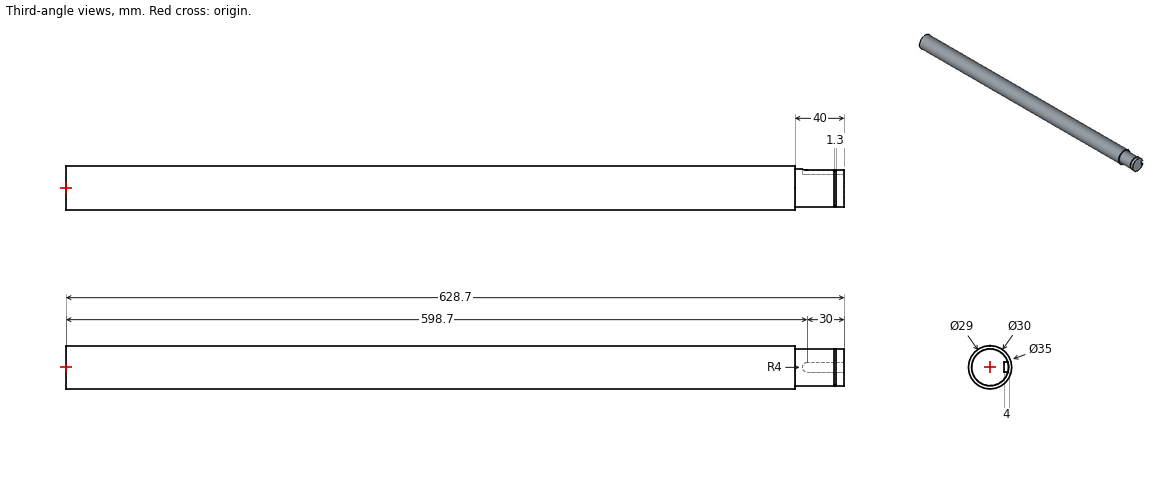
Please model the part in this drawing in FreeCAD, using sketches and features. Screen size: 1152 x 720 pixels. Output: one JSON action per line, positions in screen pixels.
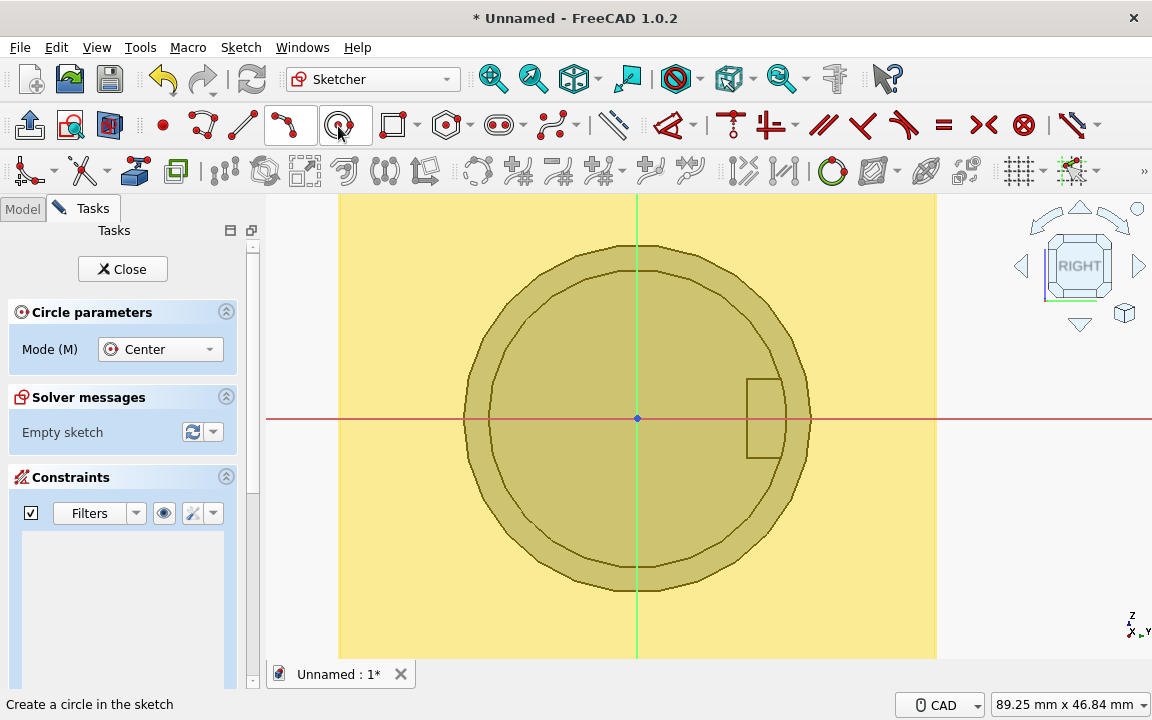
{"action": "left_click", "coordinate": [637, 419]}
{"action": "left_click", "coordinate": [743, 313]}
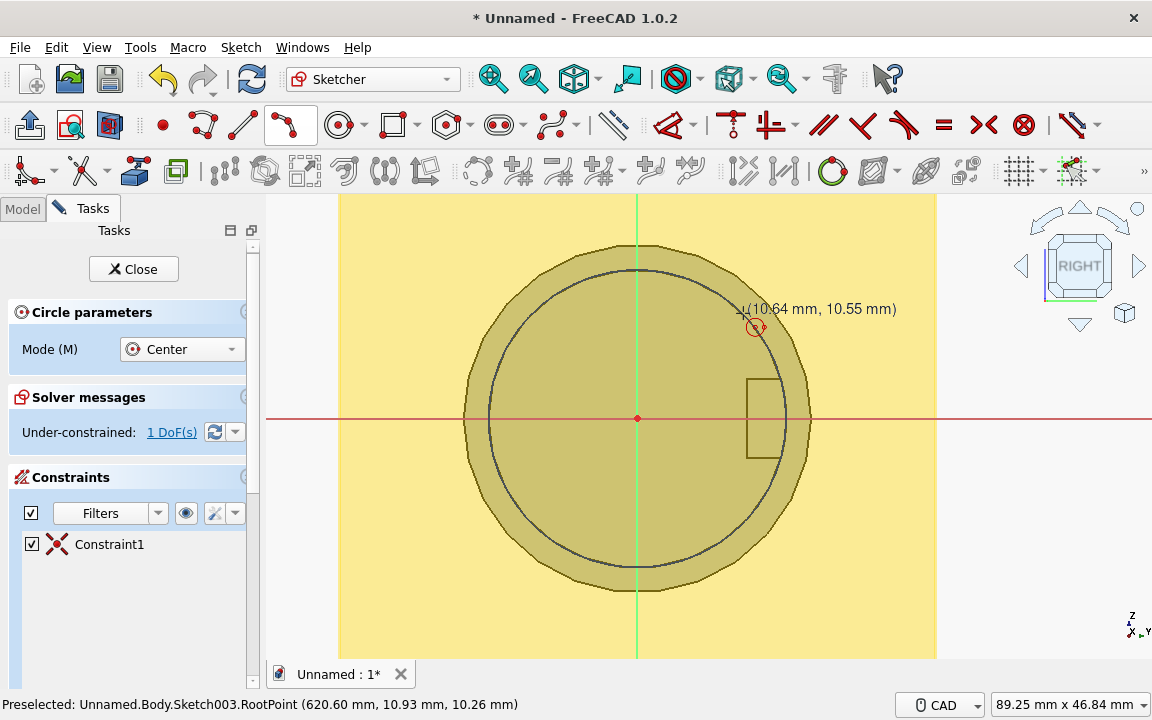
{"action": "left_click", "coordinate": [637, 419]}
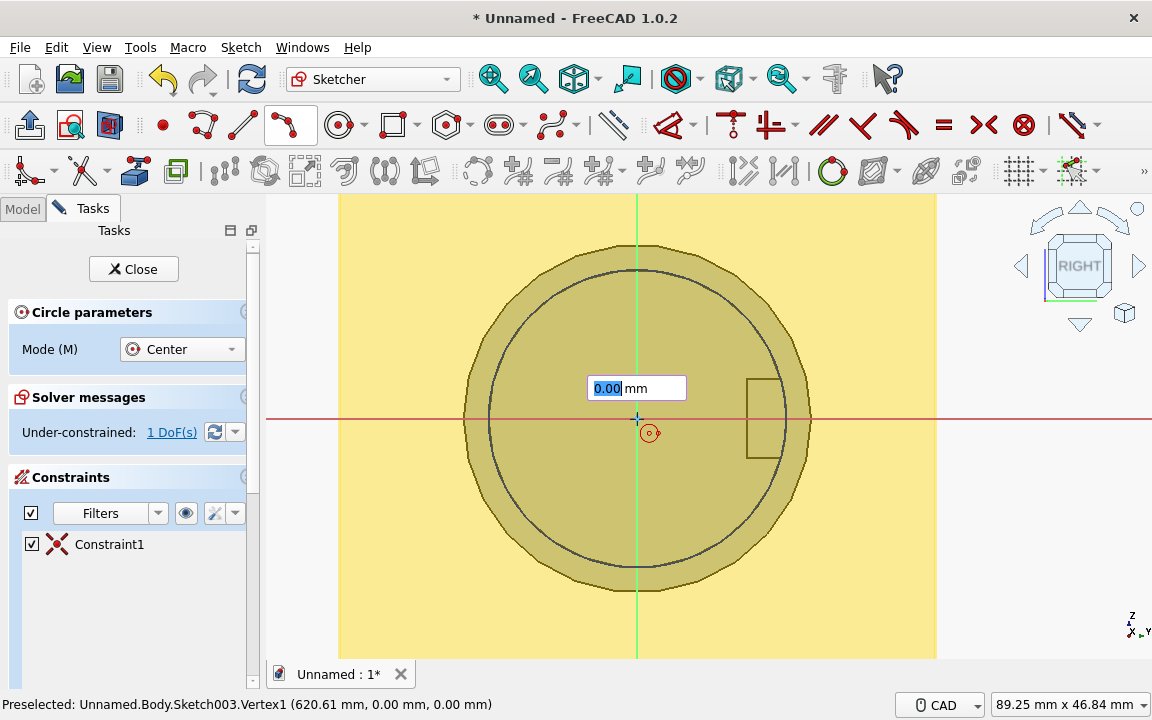
{"action": "scroll", "coordinate": [687, 284], "scroll_direction": "up", "scroll_amount": 6}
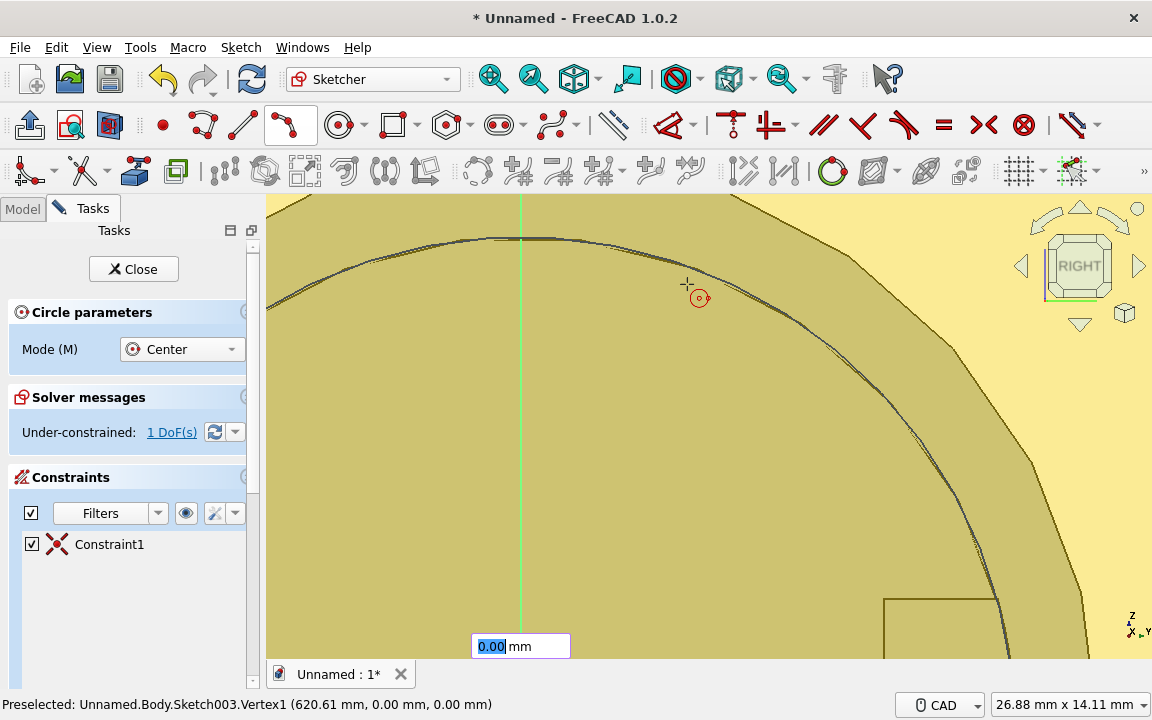
{"action": "left_click", "coordinate": [685, 282]}
{"action": "key", "text": "Escape"}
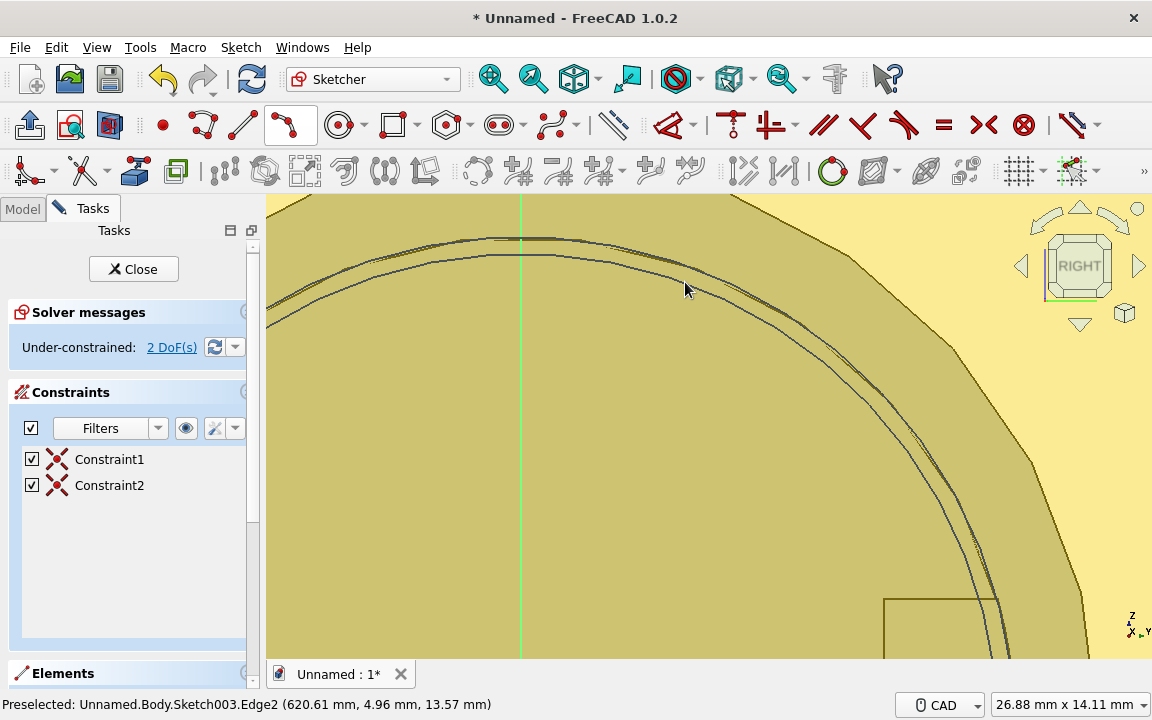
{"action": "left_click", "coordinate": [668, 126]}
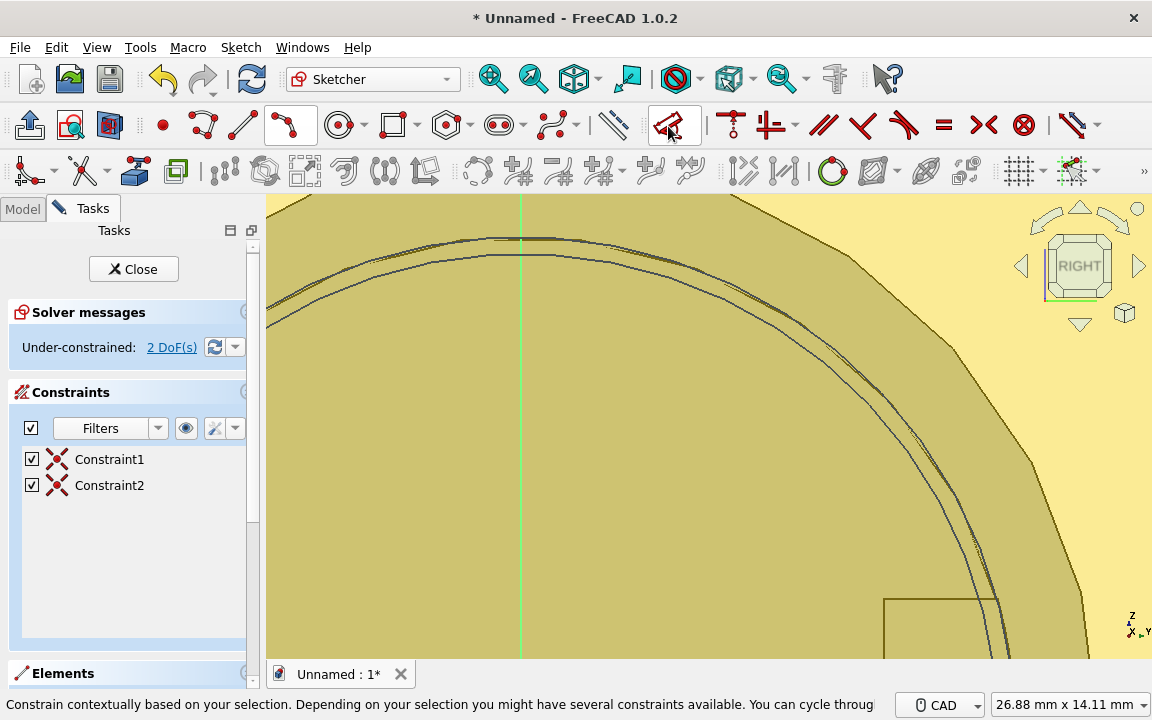
{"action": "left_click", "coordinate": [869, 381]}
{"action": "left_click", "coordinate": [892, 358]}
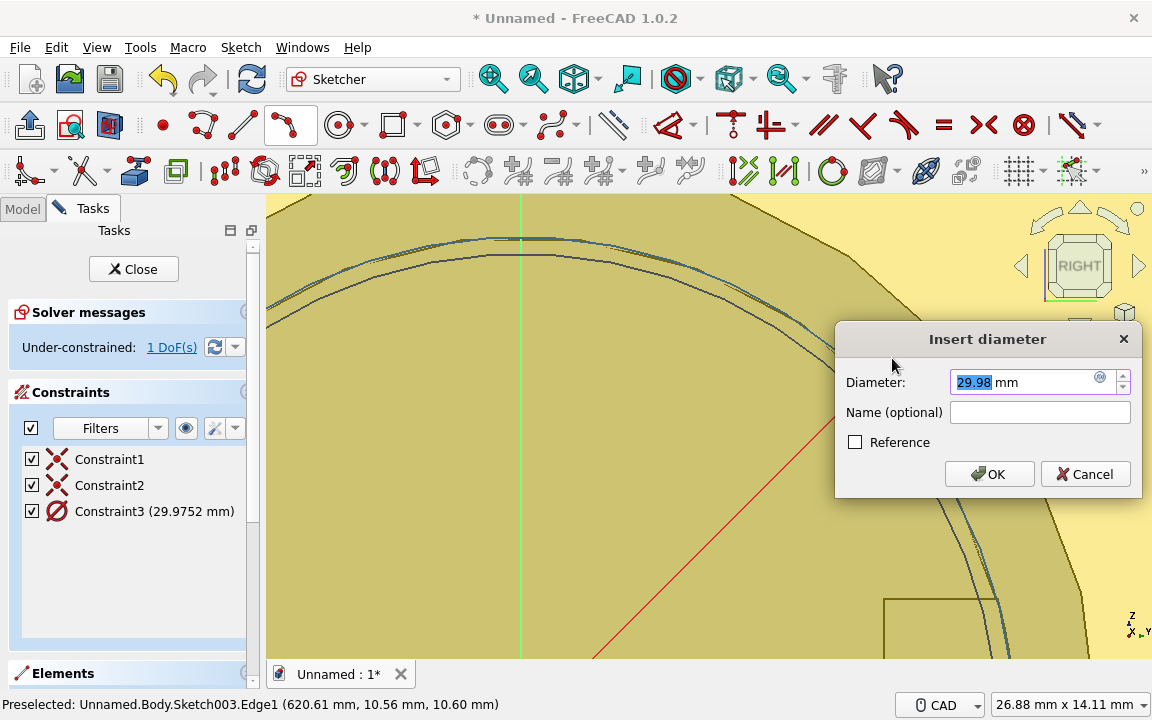
{"action": "type", "text": "30"}
{"action": "key", "text": "Return"}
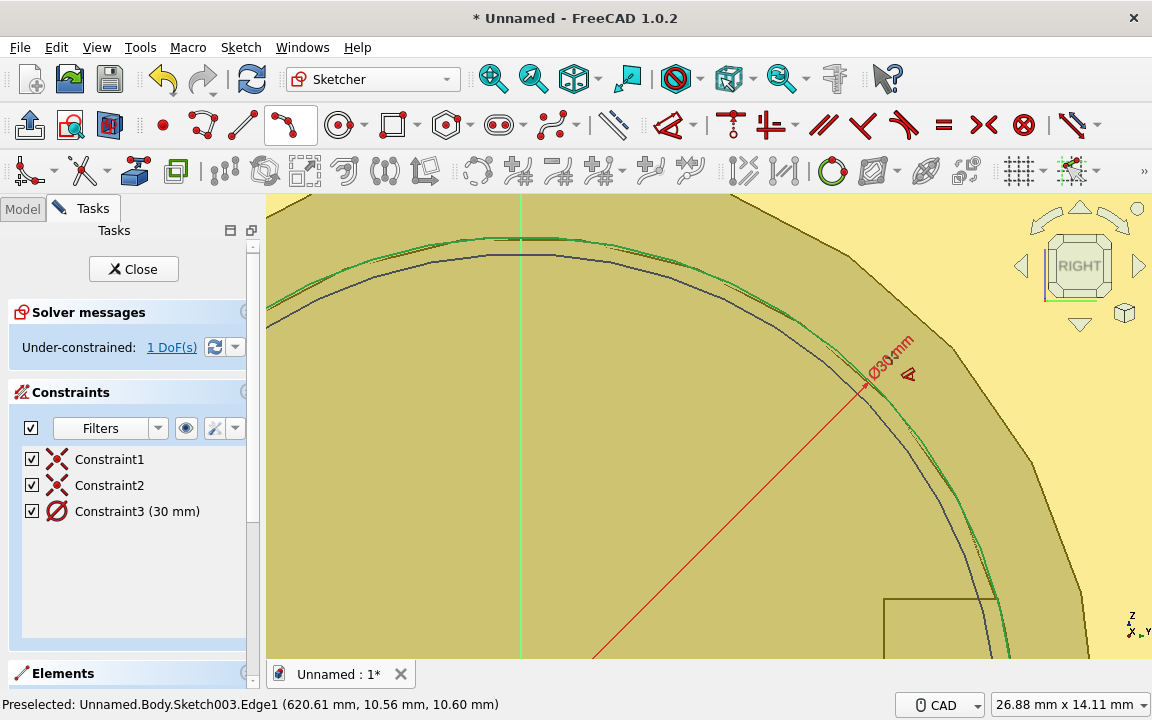
{"action": "left_click", "coordinate": [857, 393]}
{"action": "left_click", "coordinate": [663, 243]}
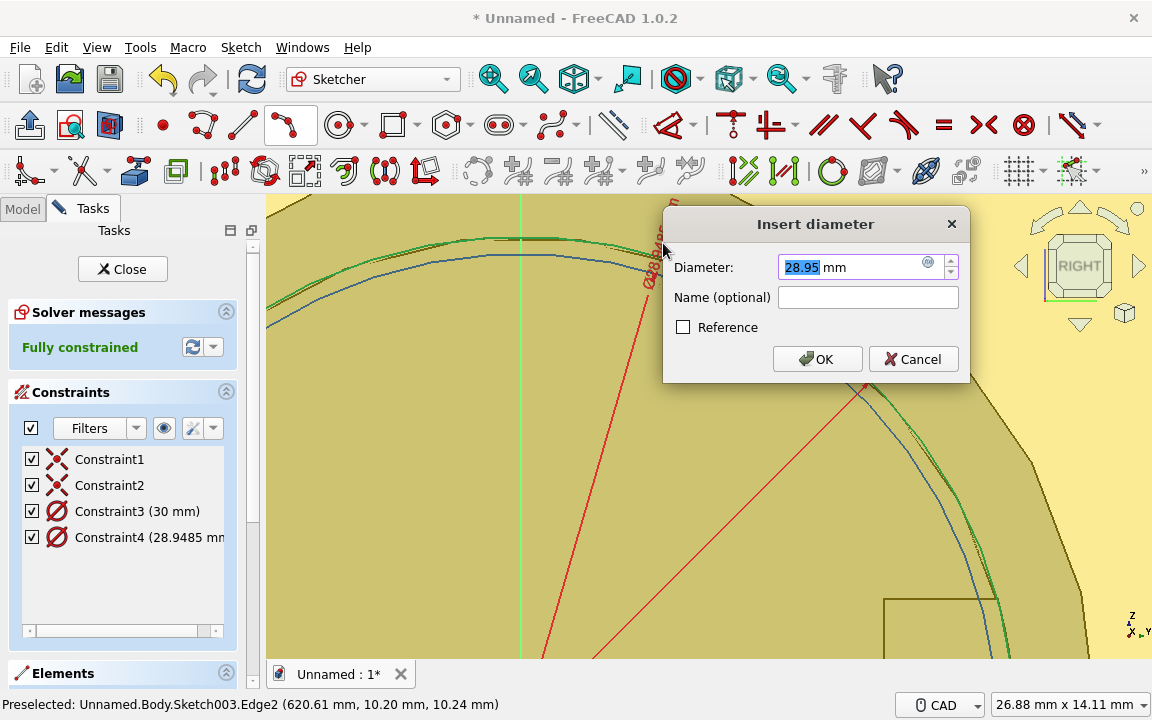
{"action": "type", "text": "29"}
{"action": "key", "text": "Return"}
{"action": "key", "text": "Escape"}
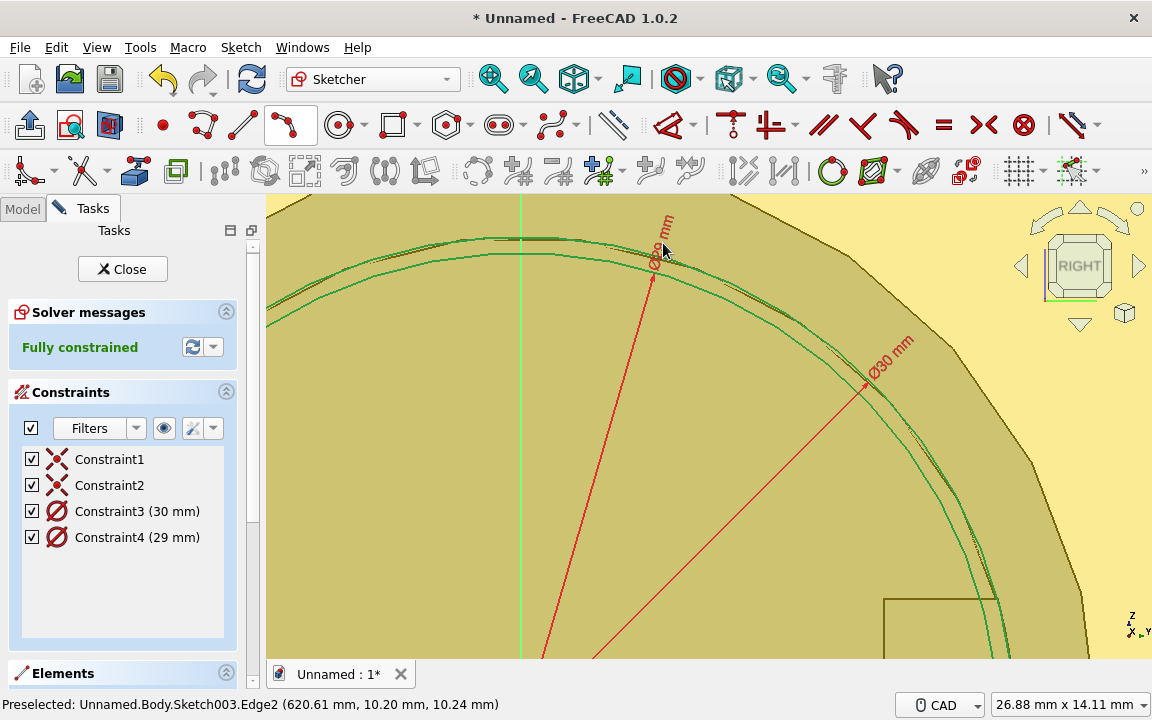
{"action": "left_click", "coordinate": [123, 269]}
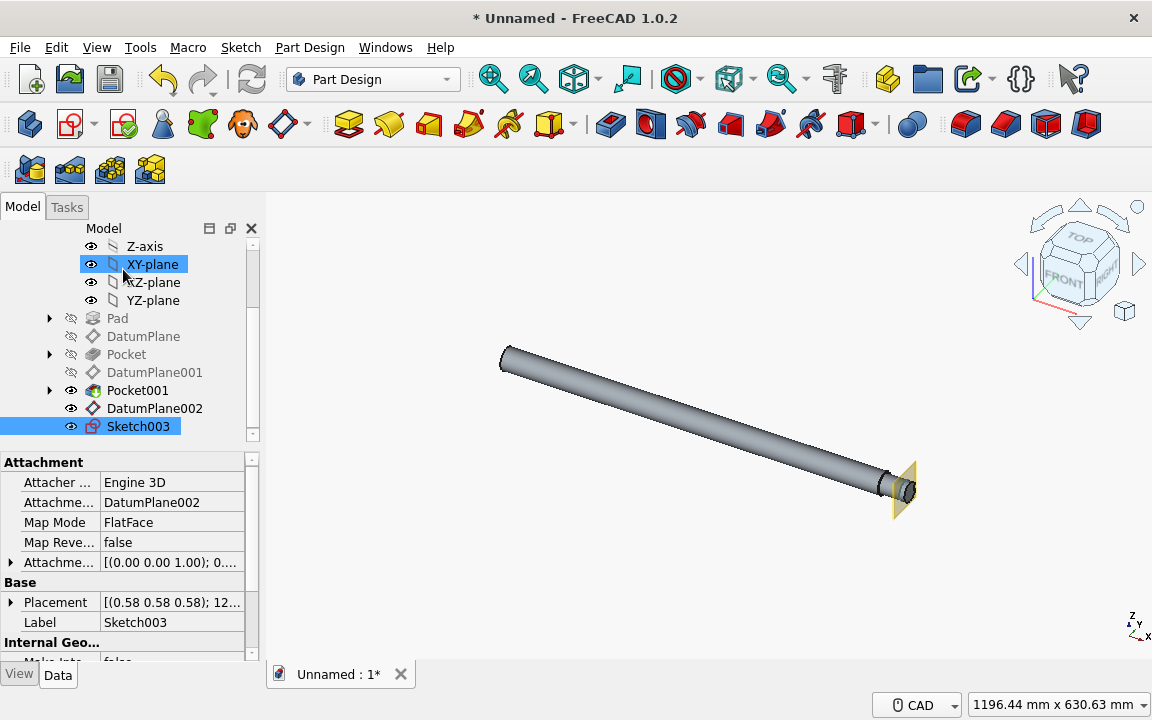
{"action": "left_click", "coordinate": [612, 124]}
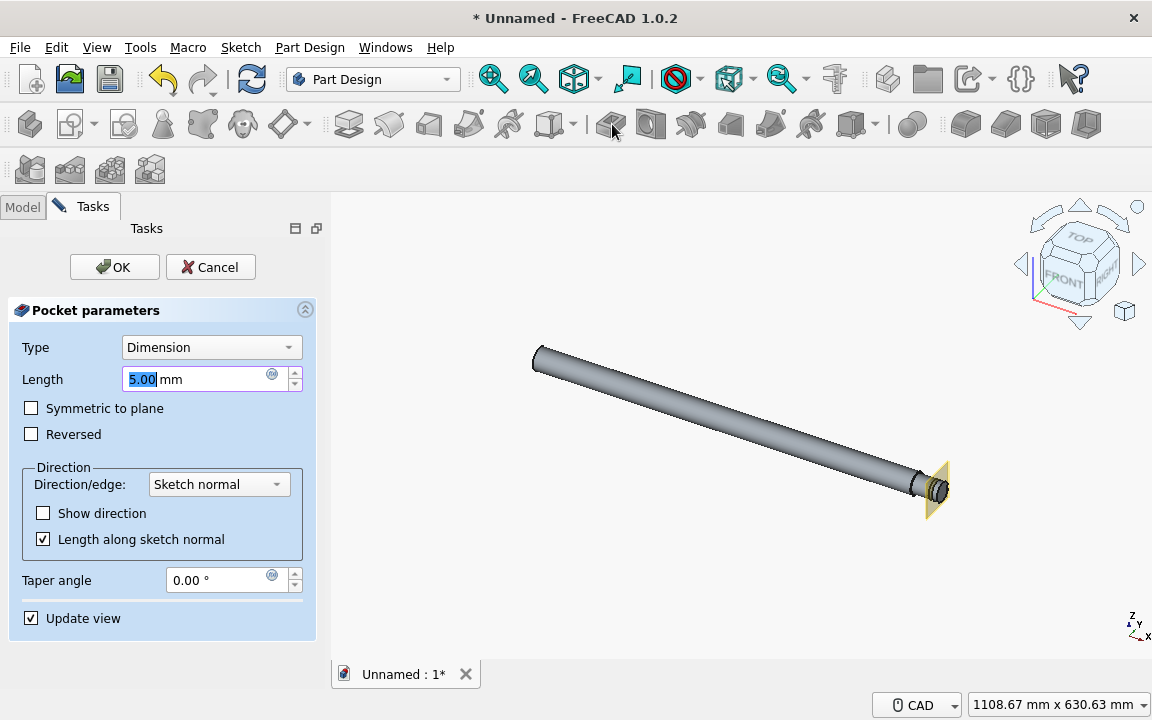
{"action": "type", "text": "1.3"}
{"action": "key", "text": "Tab"}